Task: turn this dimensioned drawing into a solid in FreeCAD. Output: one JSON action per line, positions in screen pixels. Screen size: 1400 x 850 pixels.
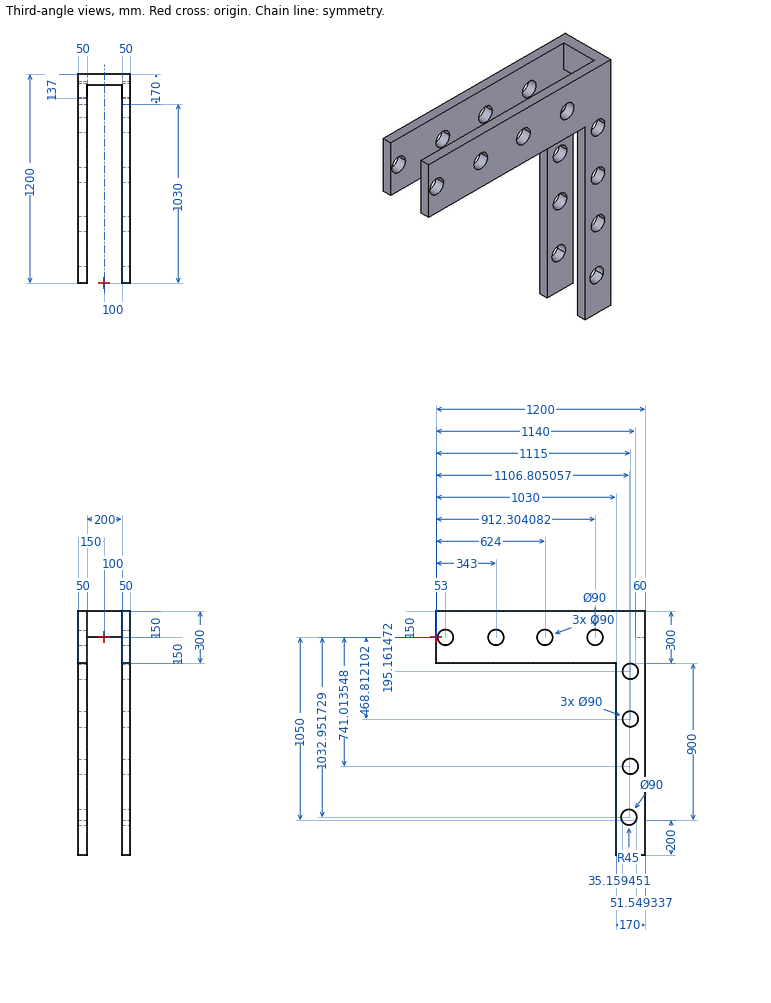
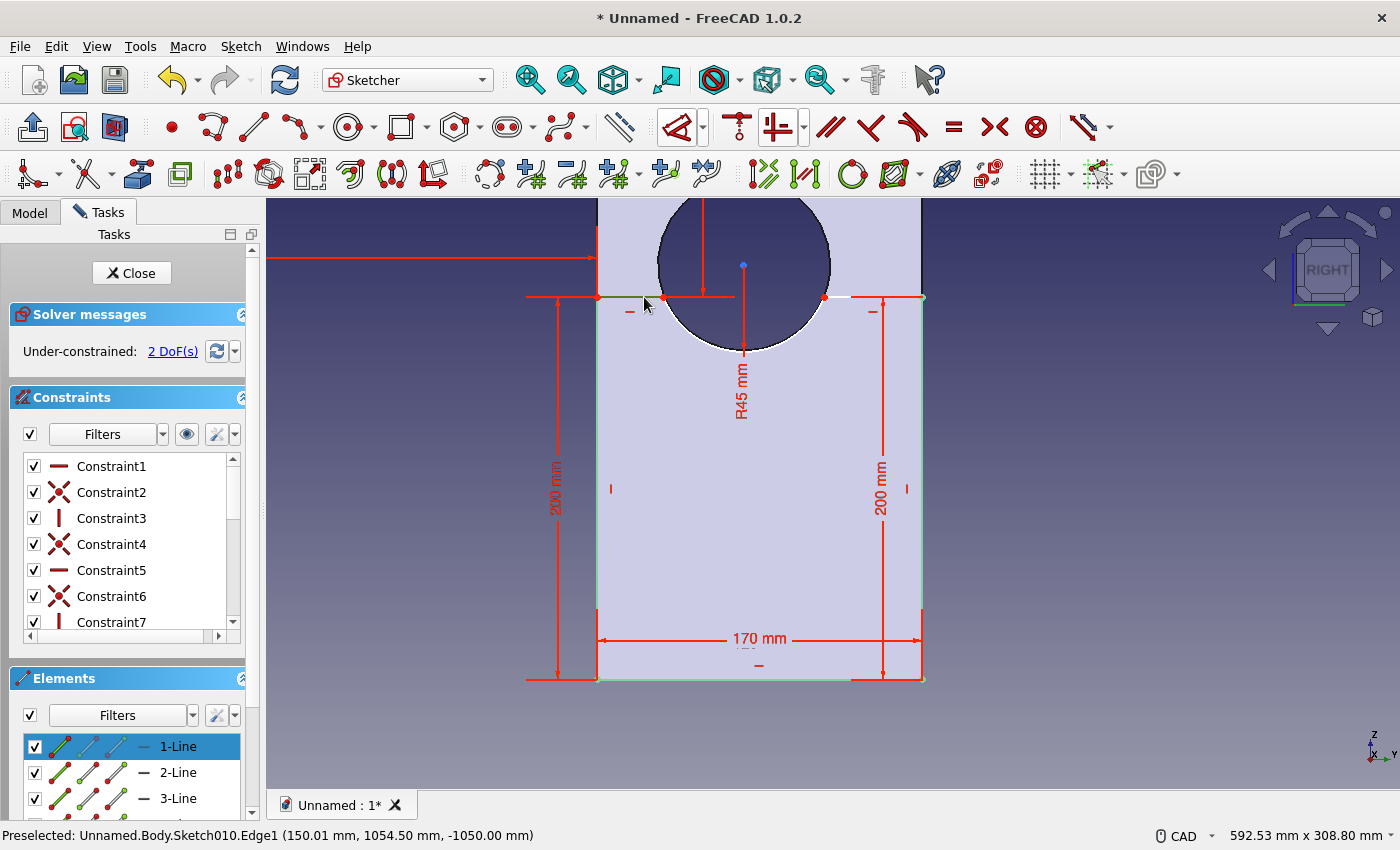
{"action": "left_click", "coordinate": [702, 128]}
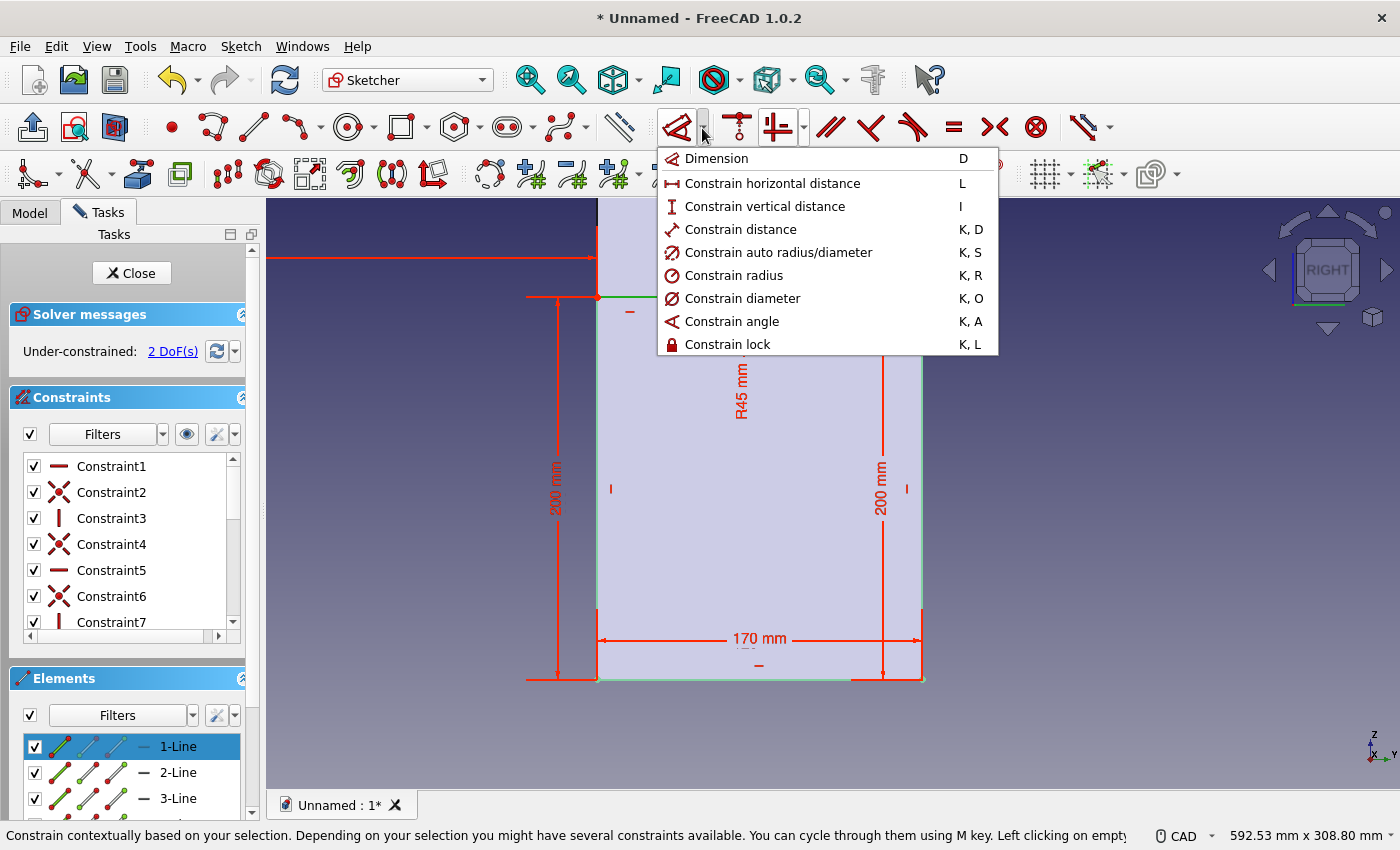
{"action": "left_click", "coordinate": [828, 184]}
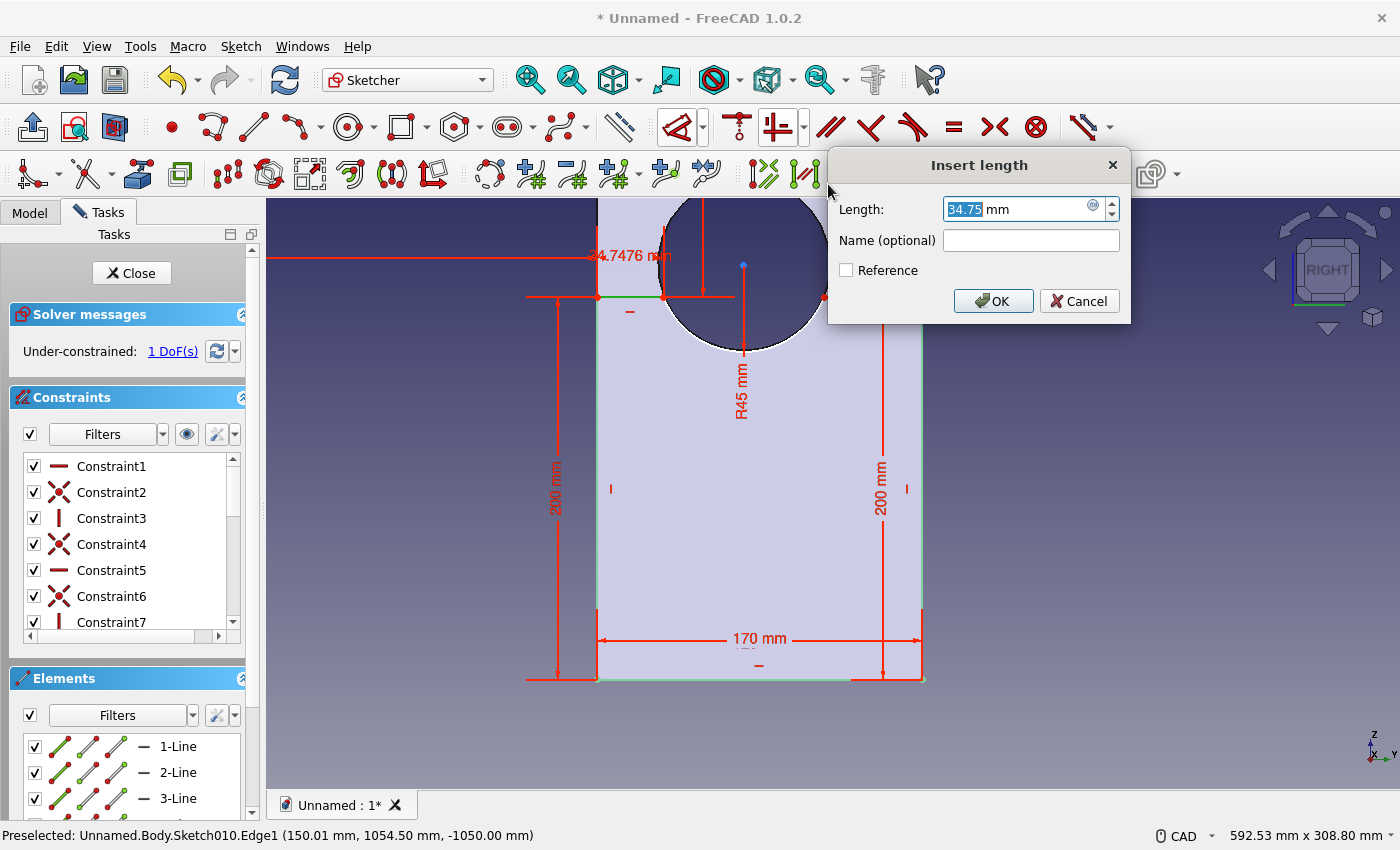
{"action": "type", "text": "35.159451"}
{"action": "key", "text": "Return"}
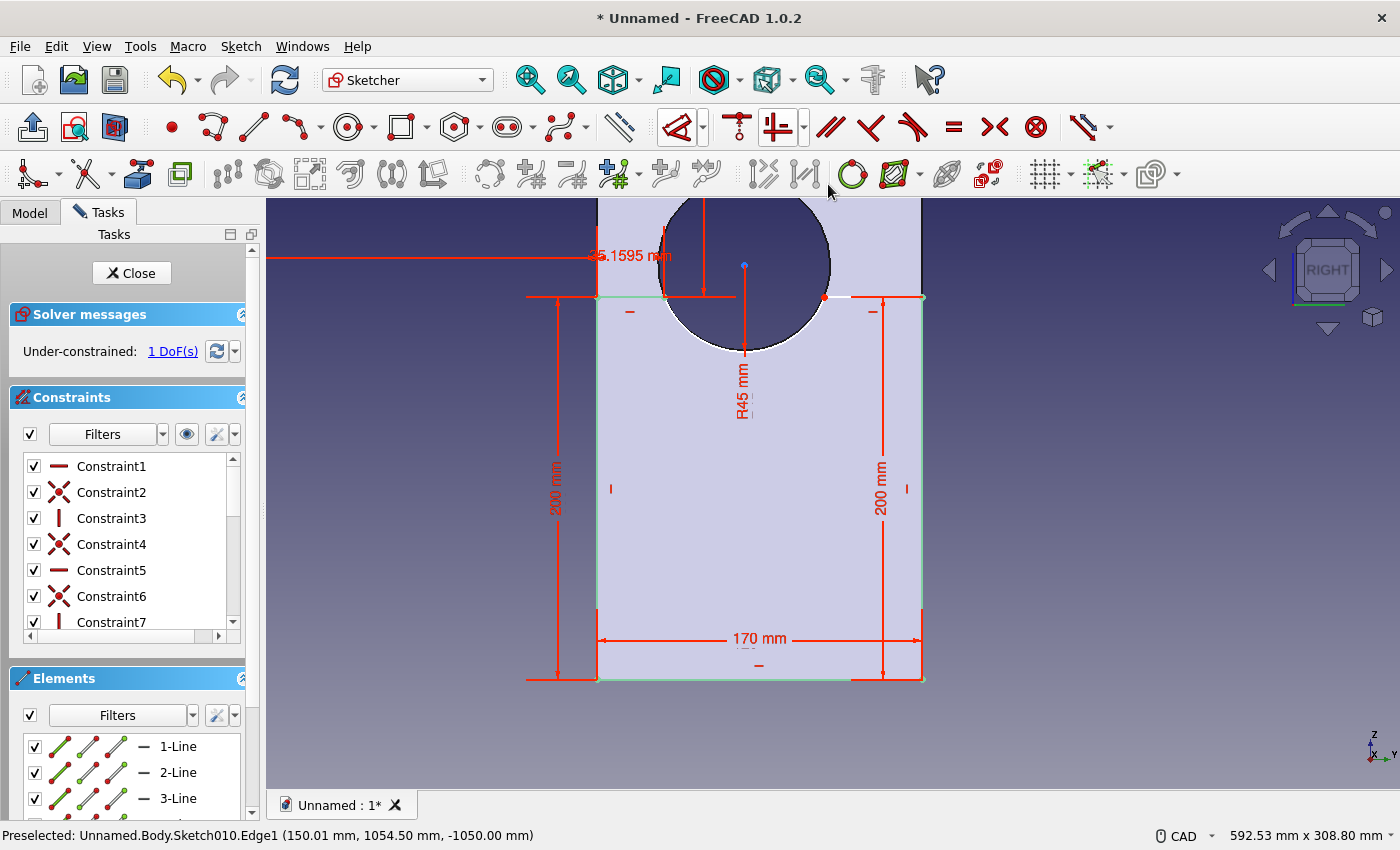
{"action": "left_click", "coordinate": [893, 297]}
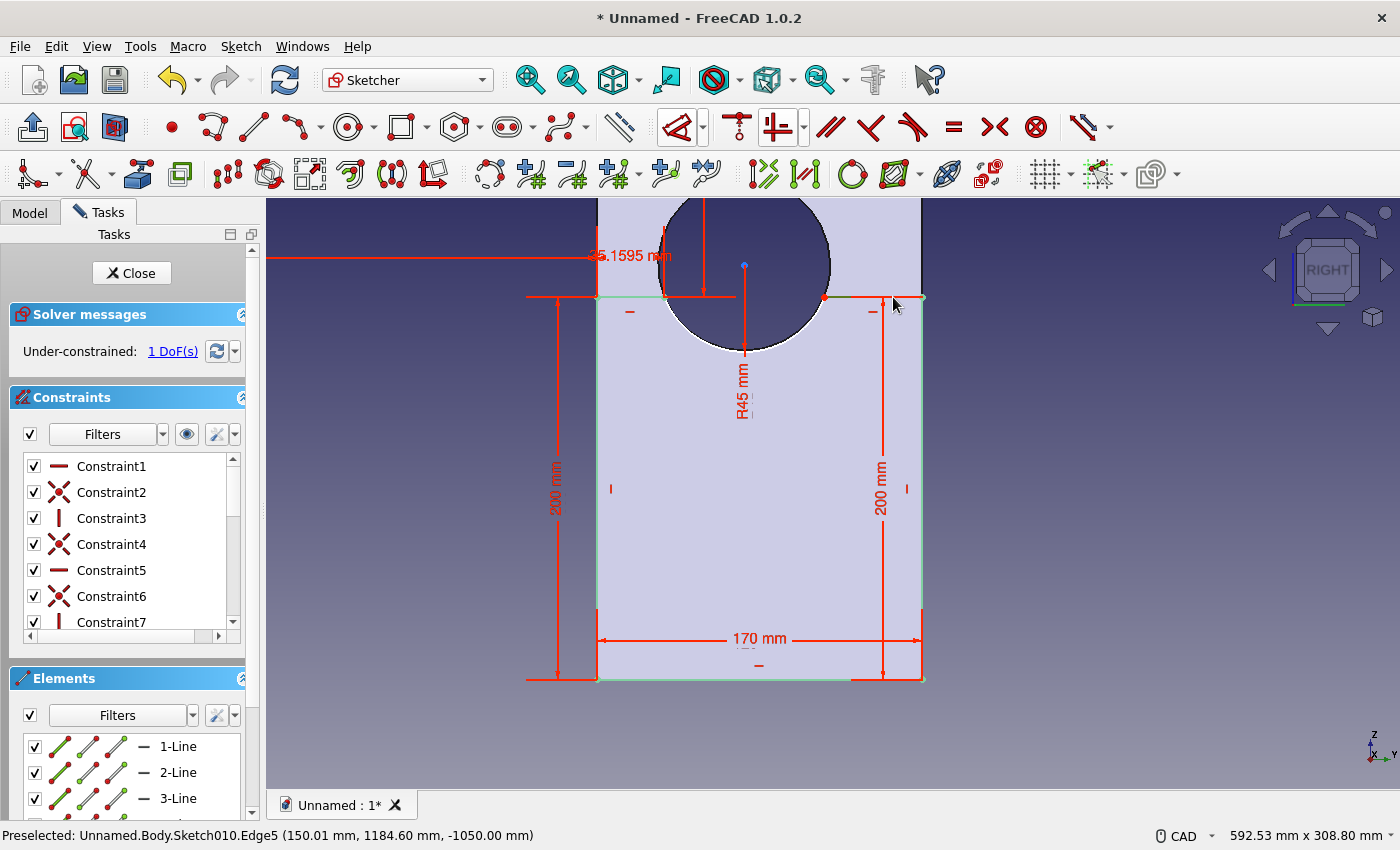
{"action": "left_click", "coordinate": [702, 128]}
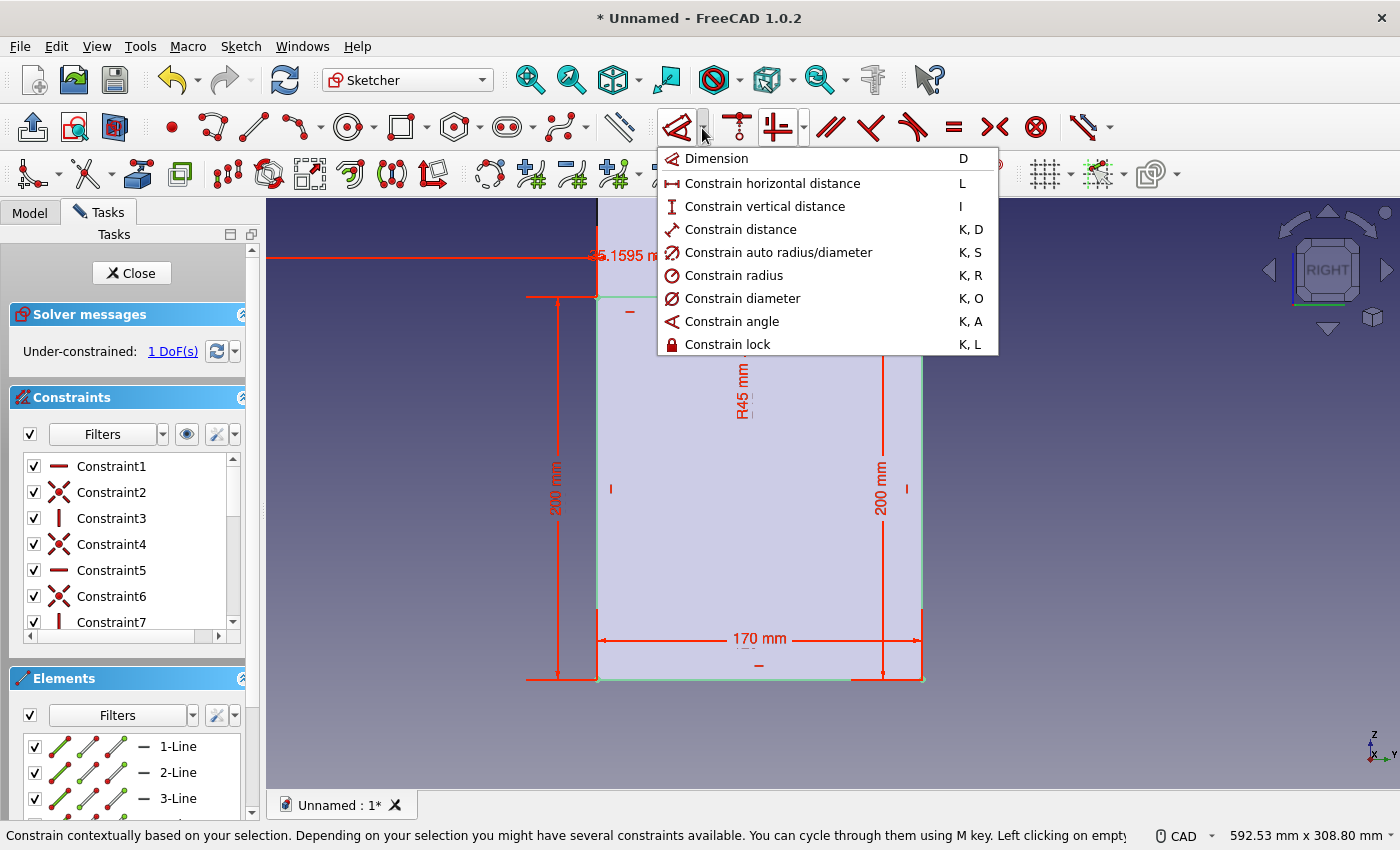
{"action": "left_click", "coordinate": [828, 184]}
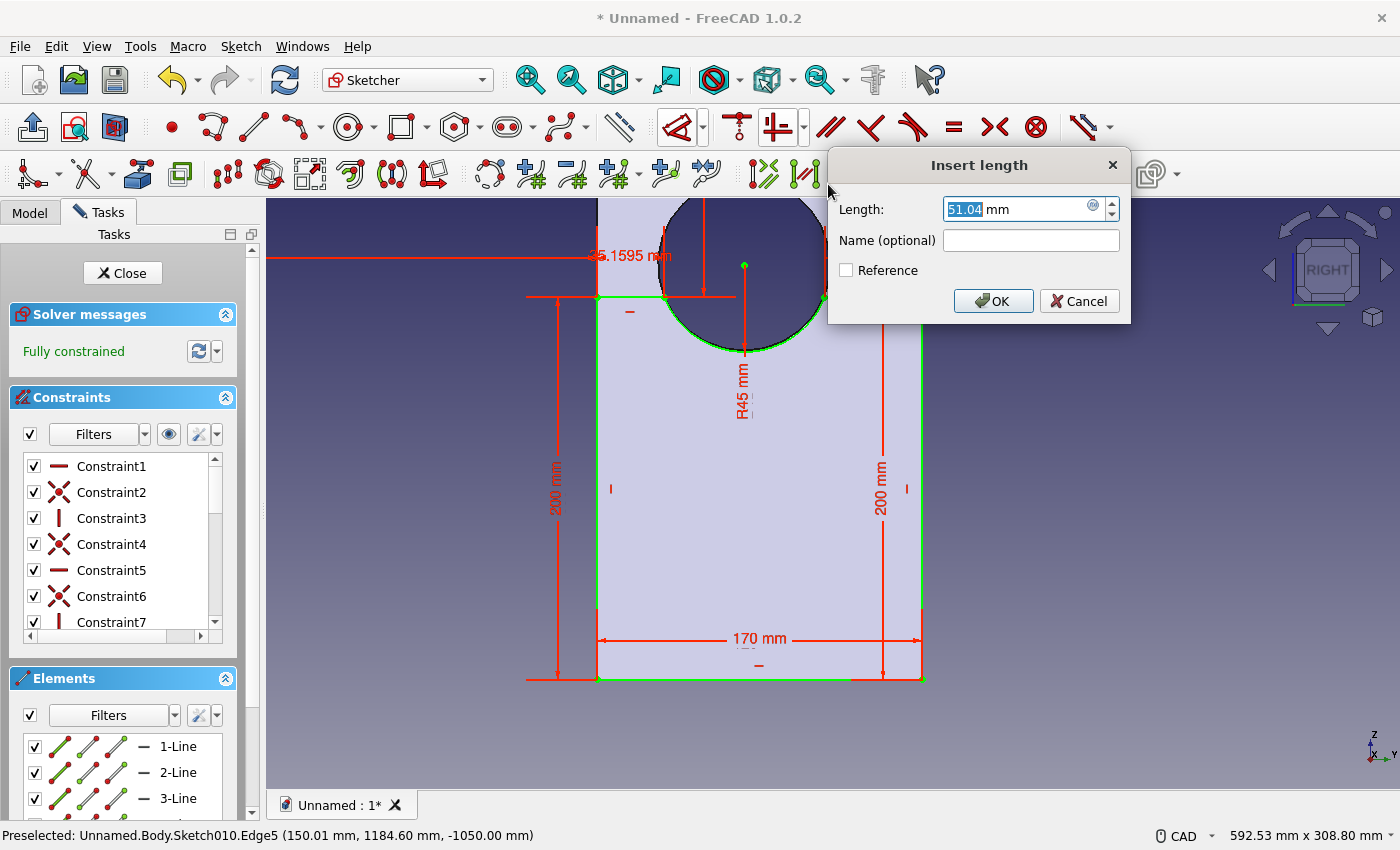
{"action": "type", "text": "51.549337"}
{"action": "key", "text": "Return"}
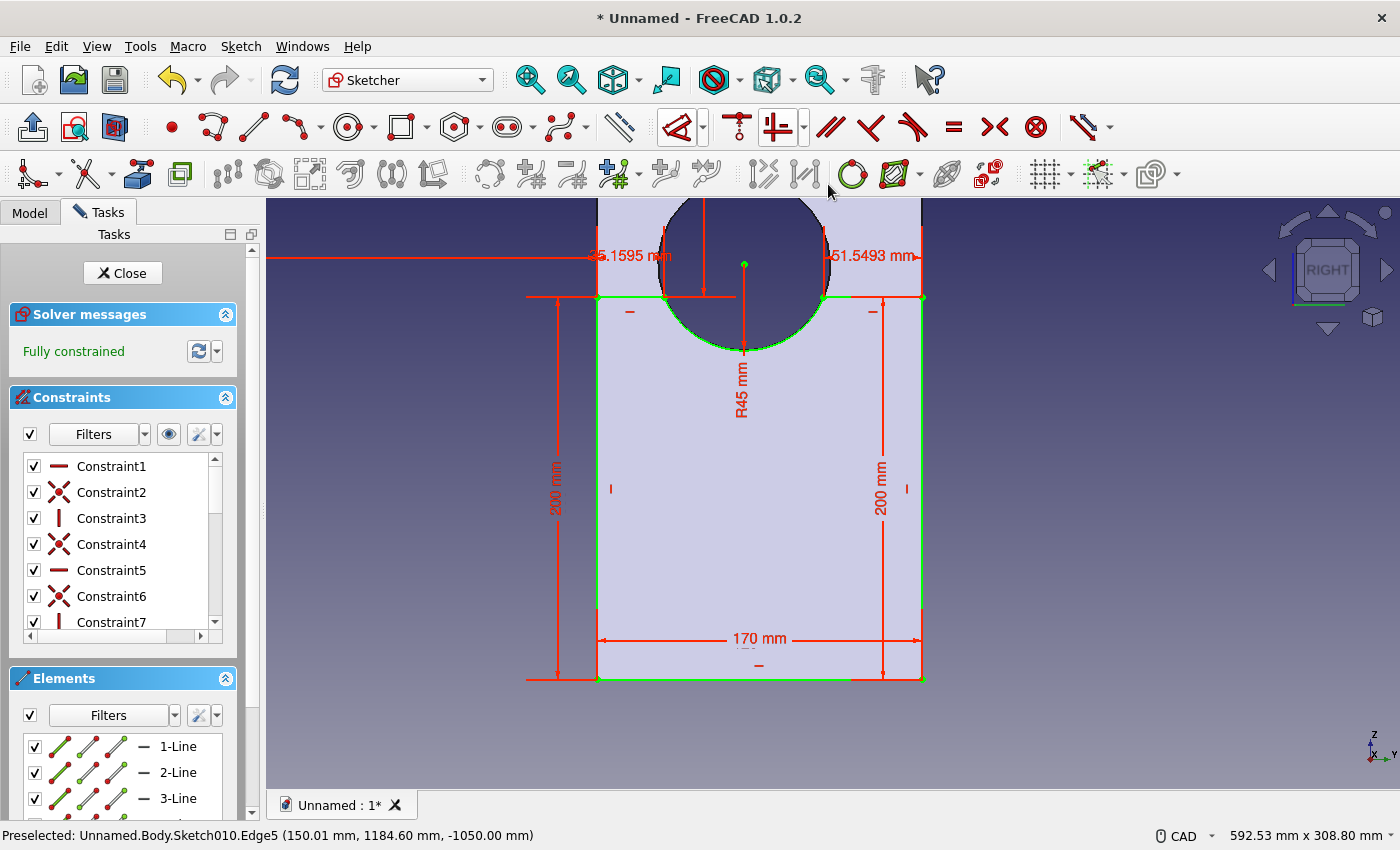
{"action": "left_click", "coordinate": [123, 273]}